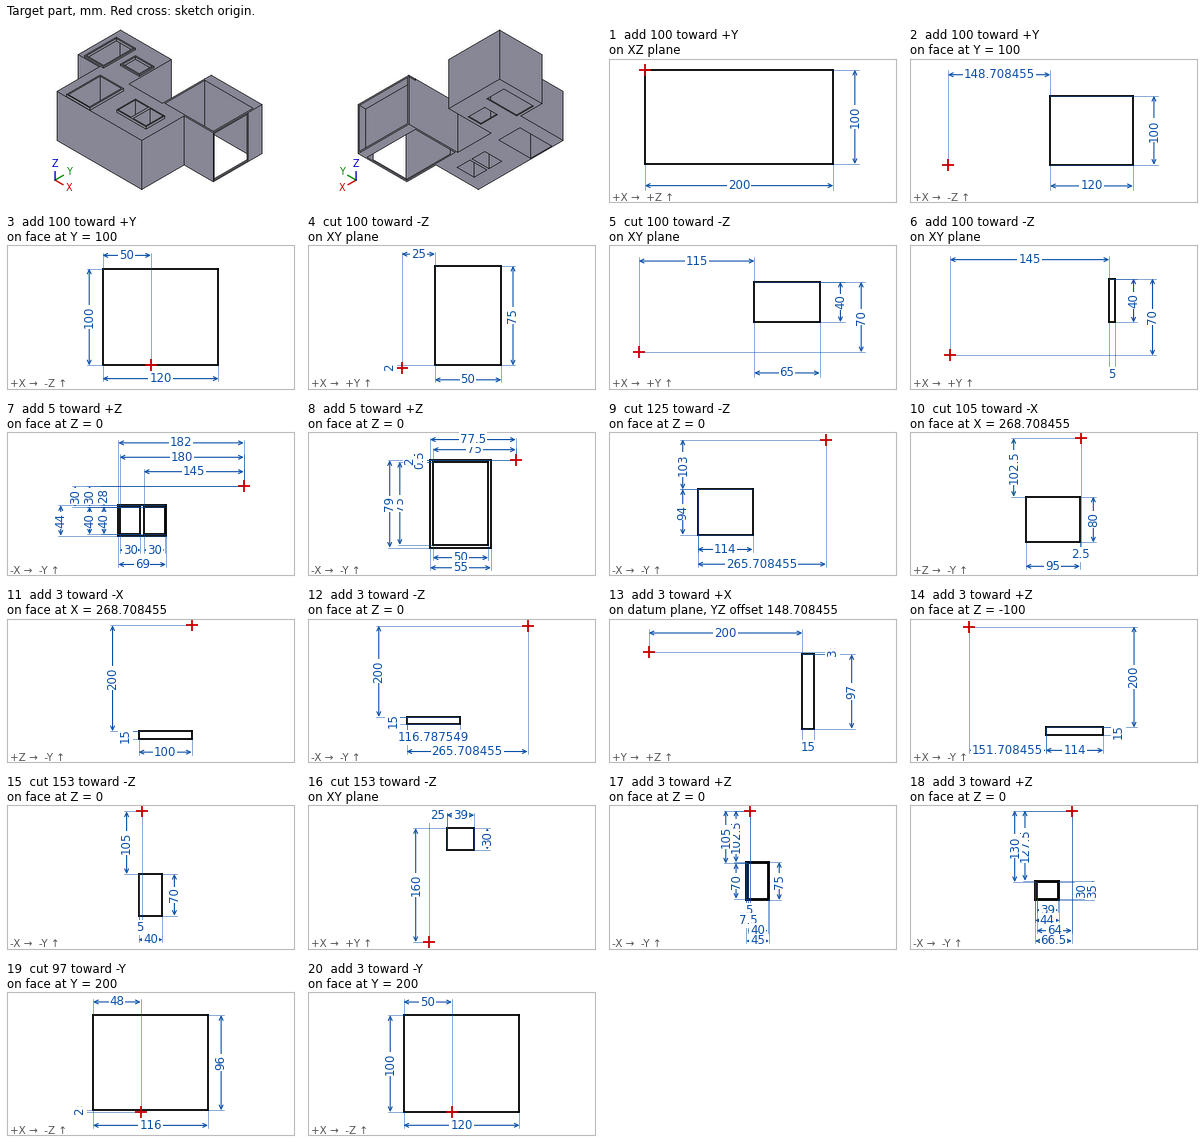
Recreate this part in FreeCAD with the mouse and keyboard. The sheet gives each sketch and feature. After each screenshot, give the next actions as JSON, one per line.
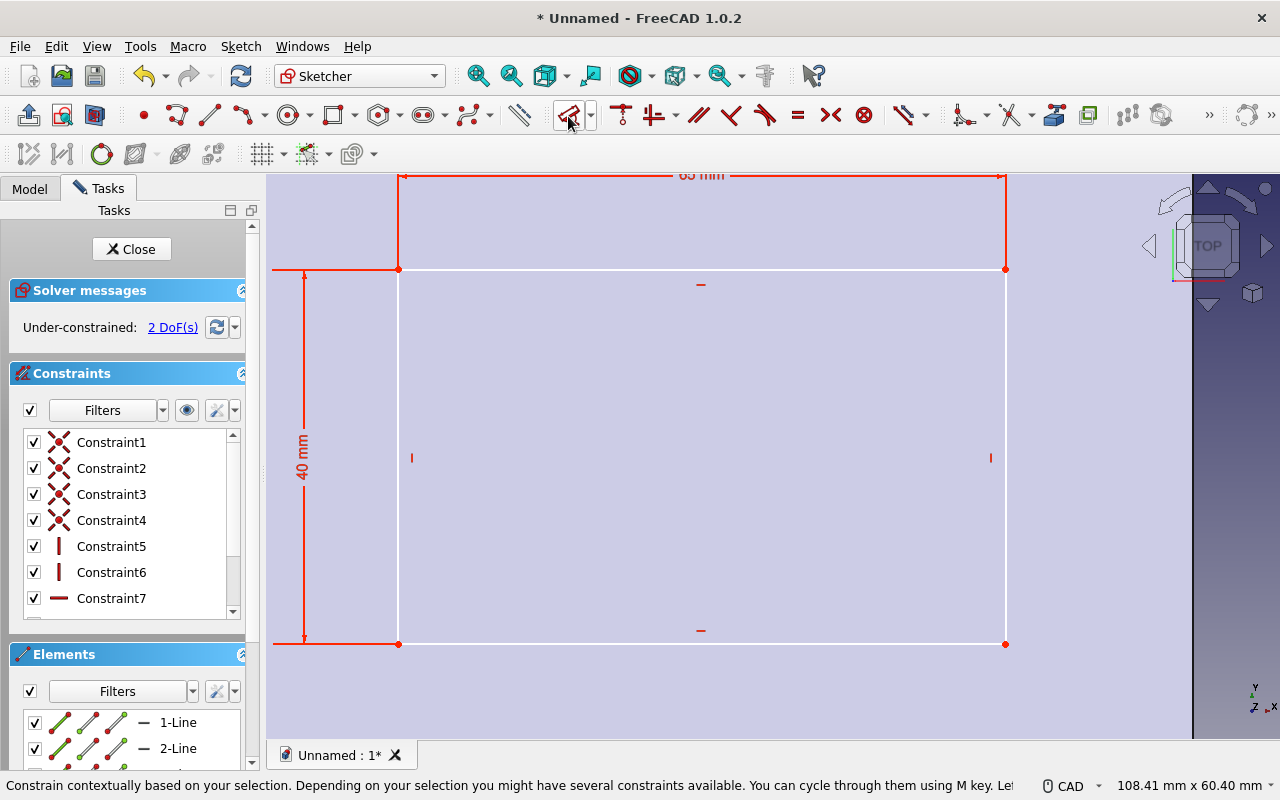
{"action": "left_click", "coordinate": [398, 270]}
{"action": "left_click", "coordinate": [432, 491]}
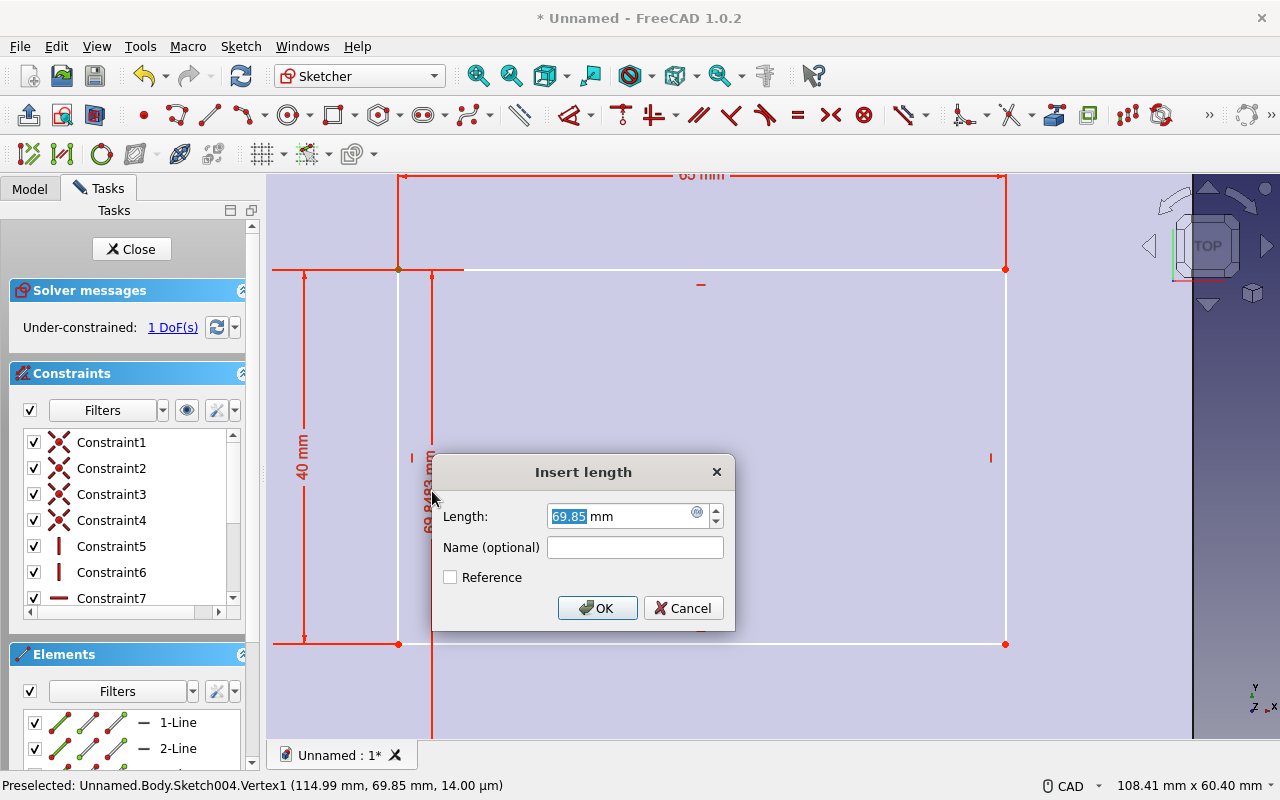
{"action": "type", "text": "70"}
{"action": "key", "text": "Return"}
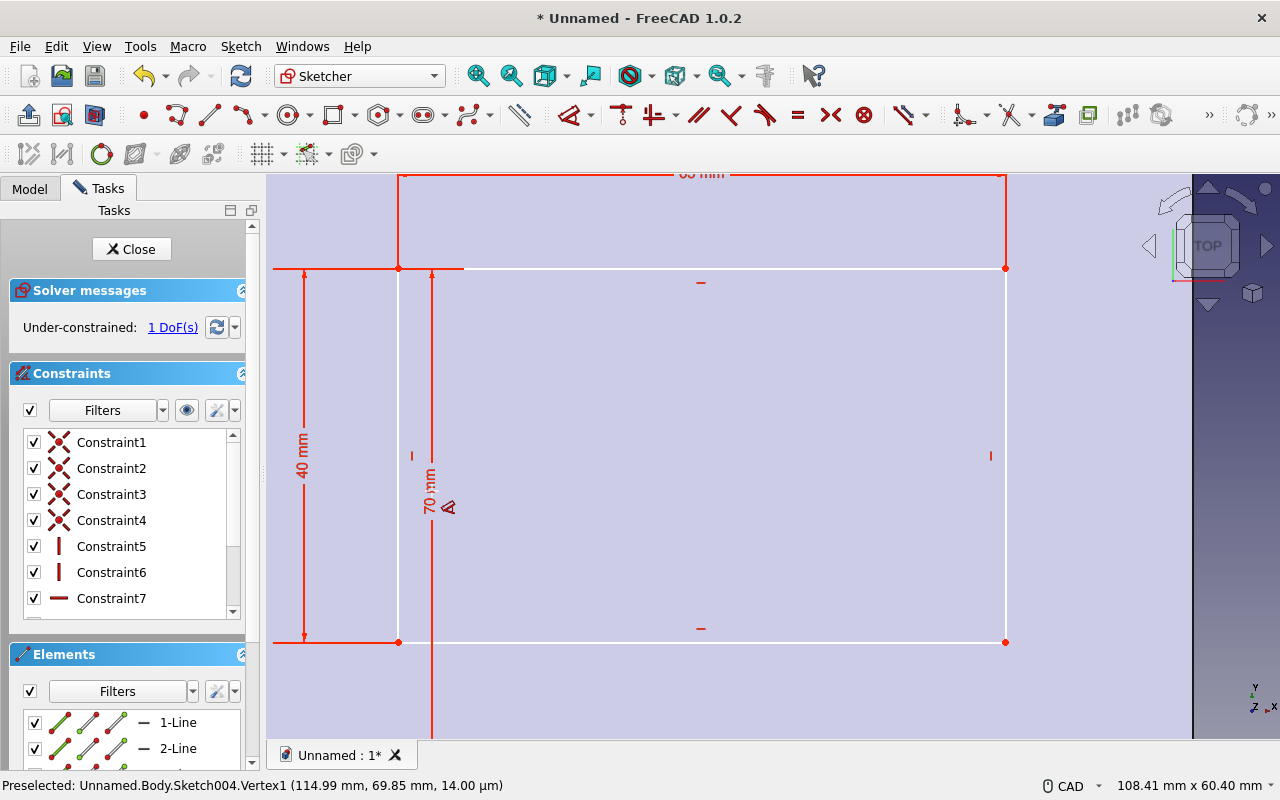
{"action": "left_click", "coordinate": [398, 269]}
{"action": "left_click", "coordinate": [346, 235]}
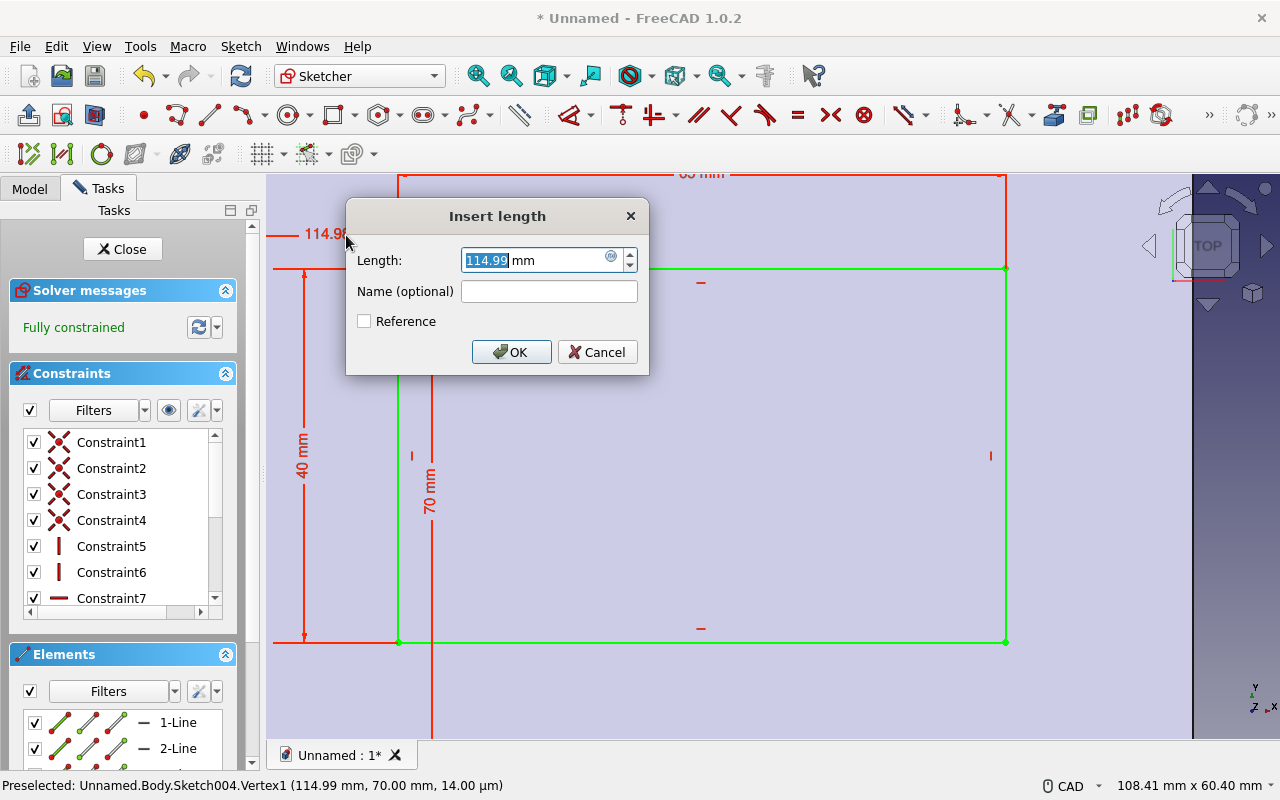
{"action": "type", "text": "115"}
{"action": "key", "text": "Return"}
{"action": "key", "text": "Escape"}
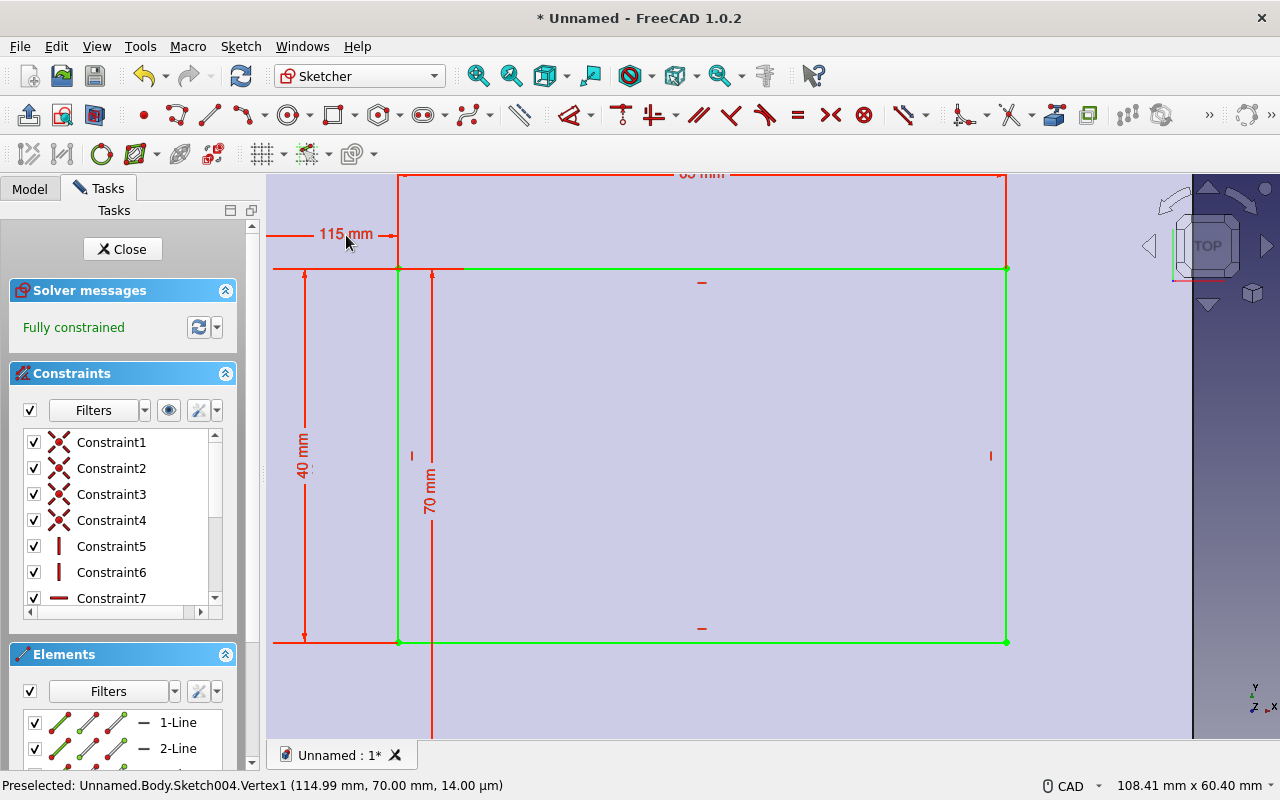
{"action": "left_click", "coordinate": [123, 249]}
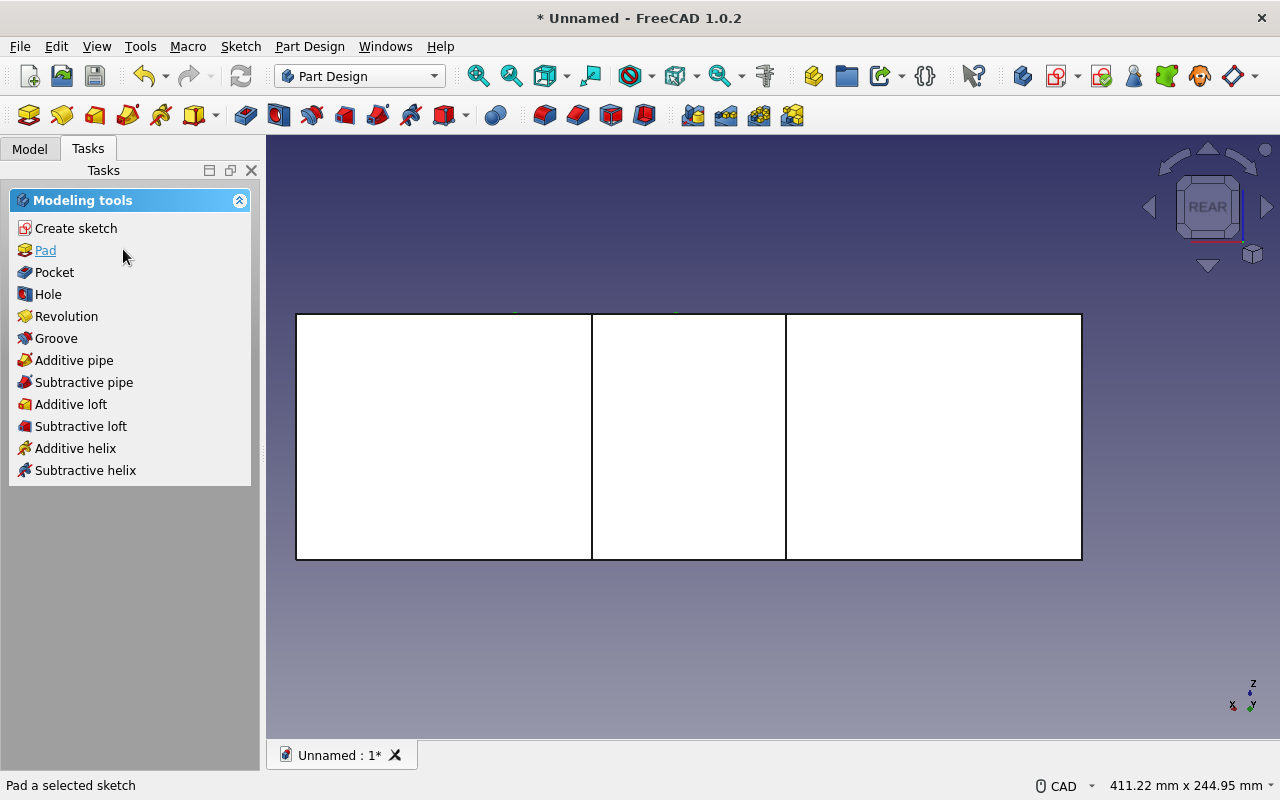
{"action": "left_click", "coordinate": [246, 116]}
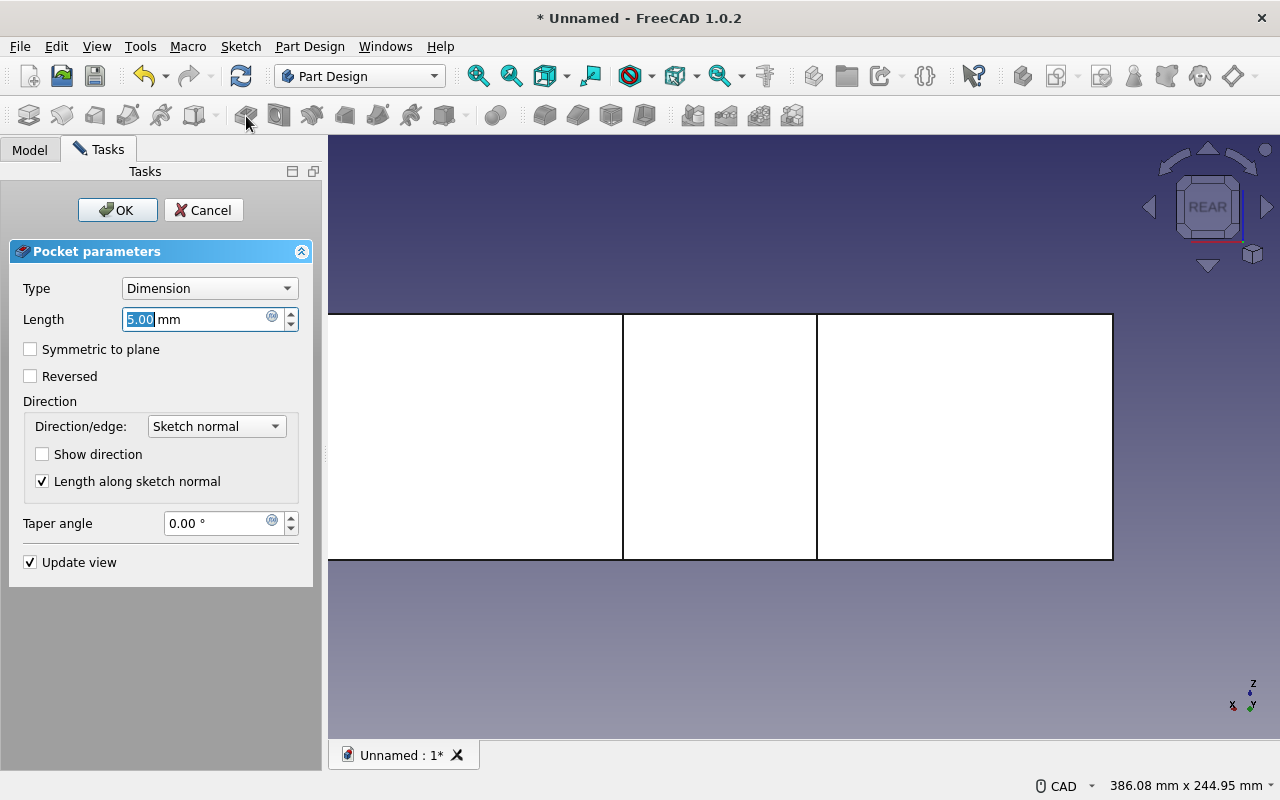
{"action": "type", "text": "100"}
{"action": "key", "text": "Tab"}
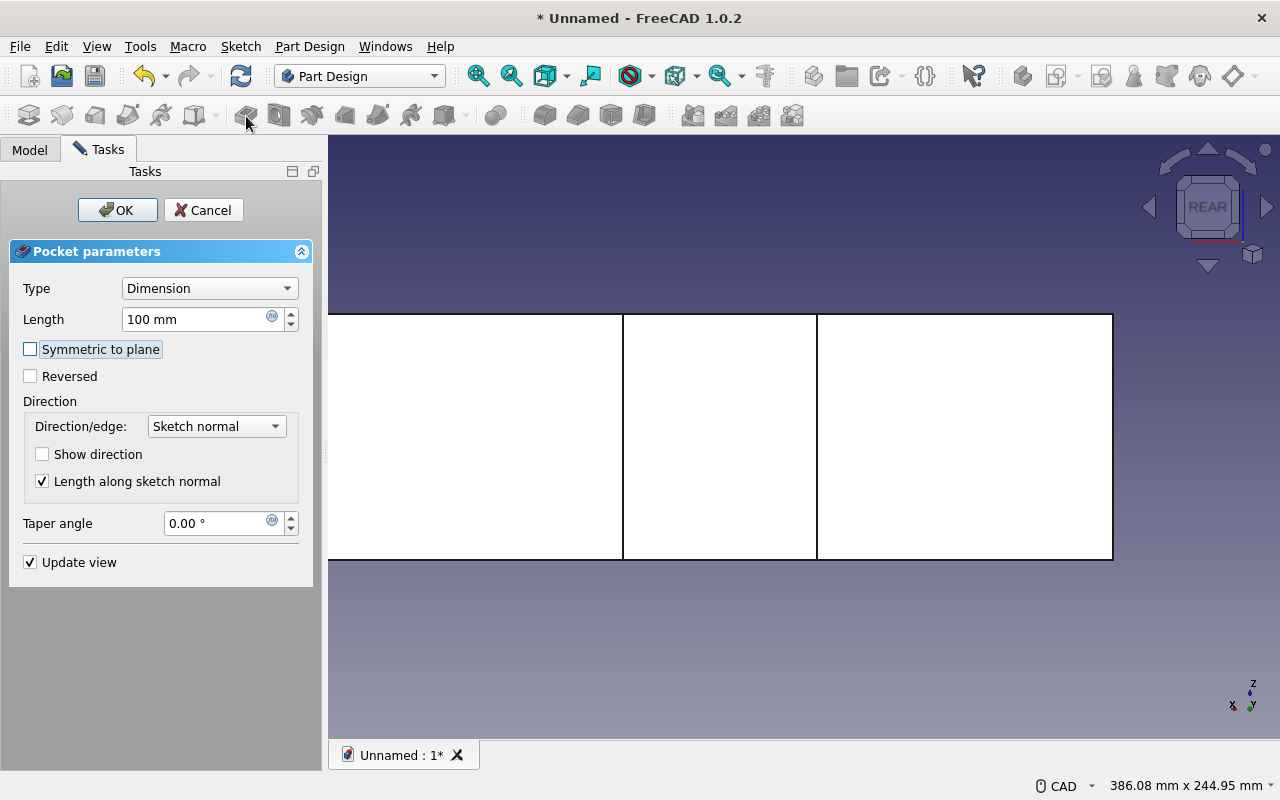
{"action": "left_click", "coordinate": [118, 210]}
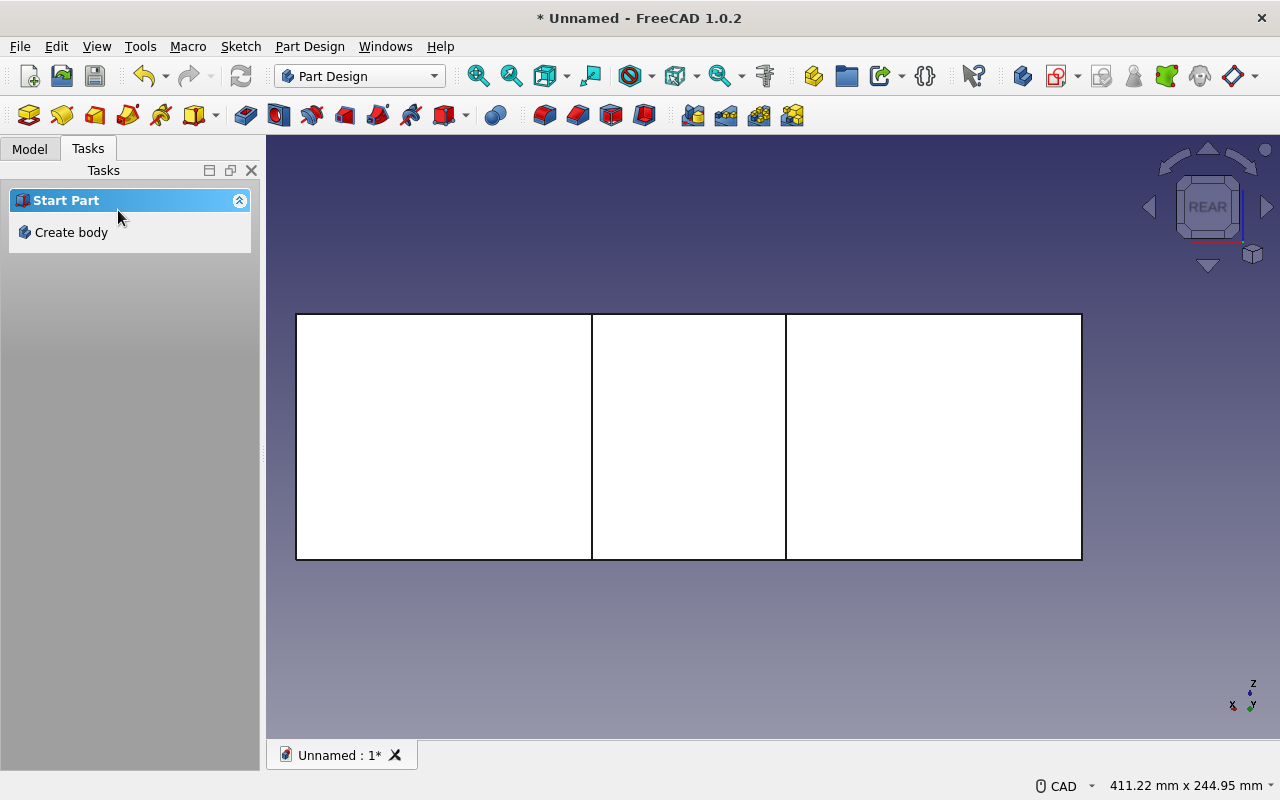
{"action": "left_click", "coordinate": [1056, 76]}